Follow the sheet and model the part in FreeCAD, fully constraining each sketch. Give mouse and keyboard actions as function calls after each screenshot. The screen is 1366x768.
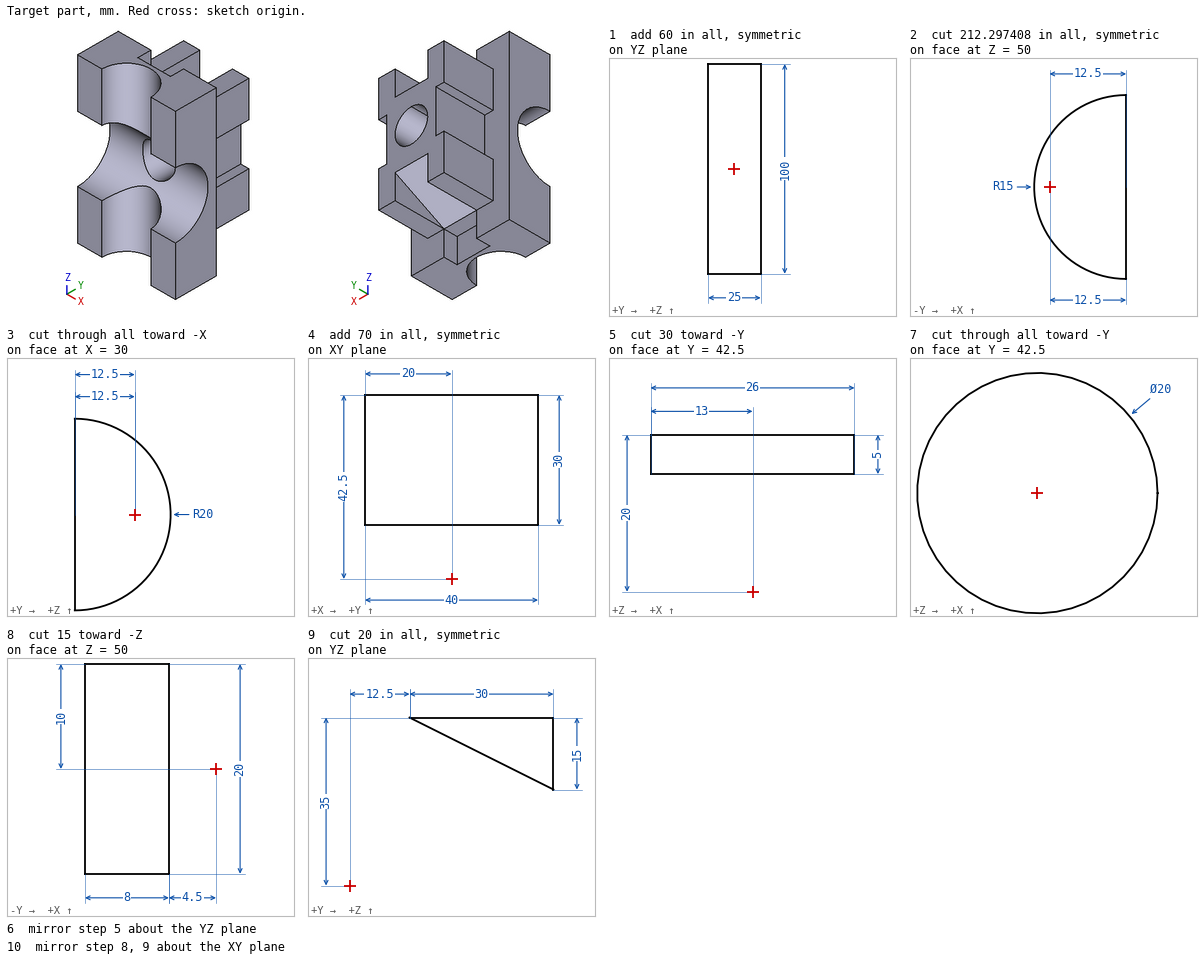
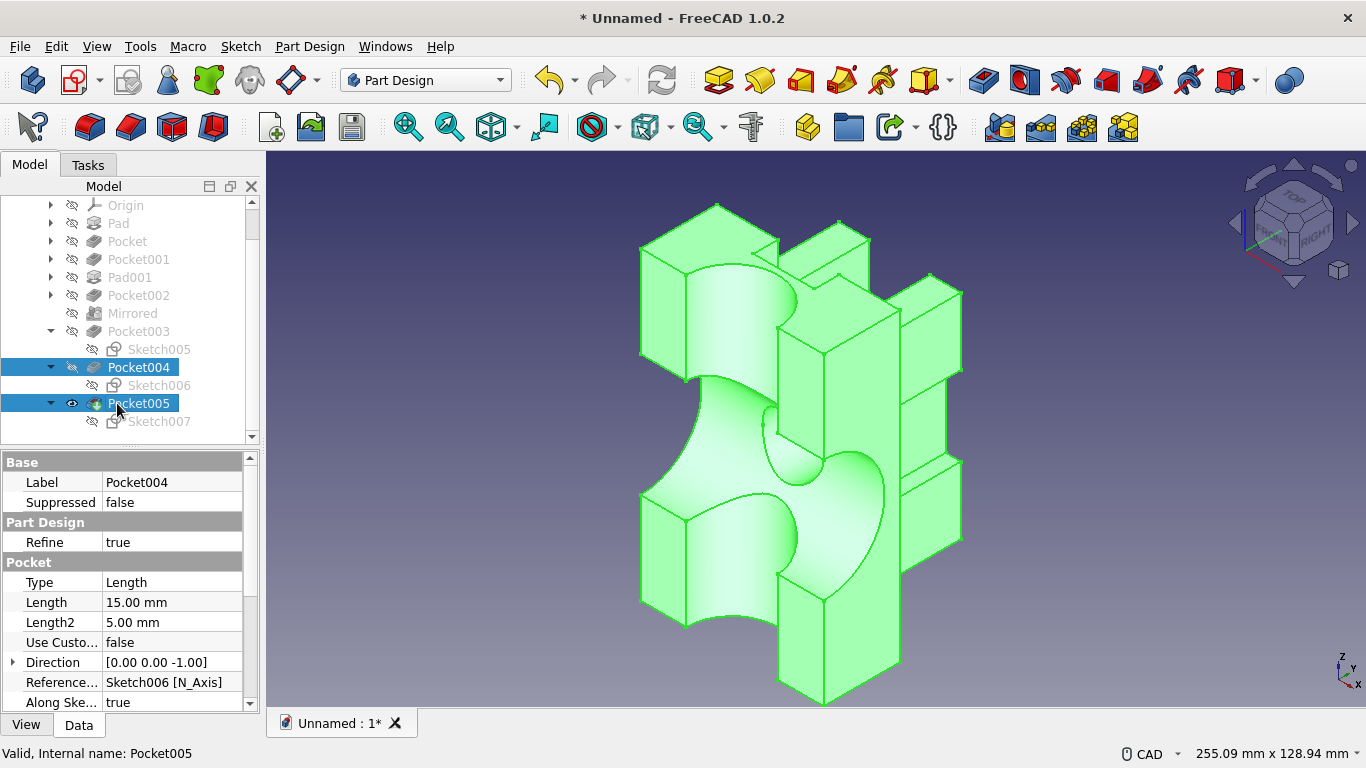
click(1000, 128)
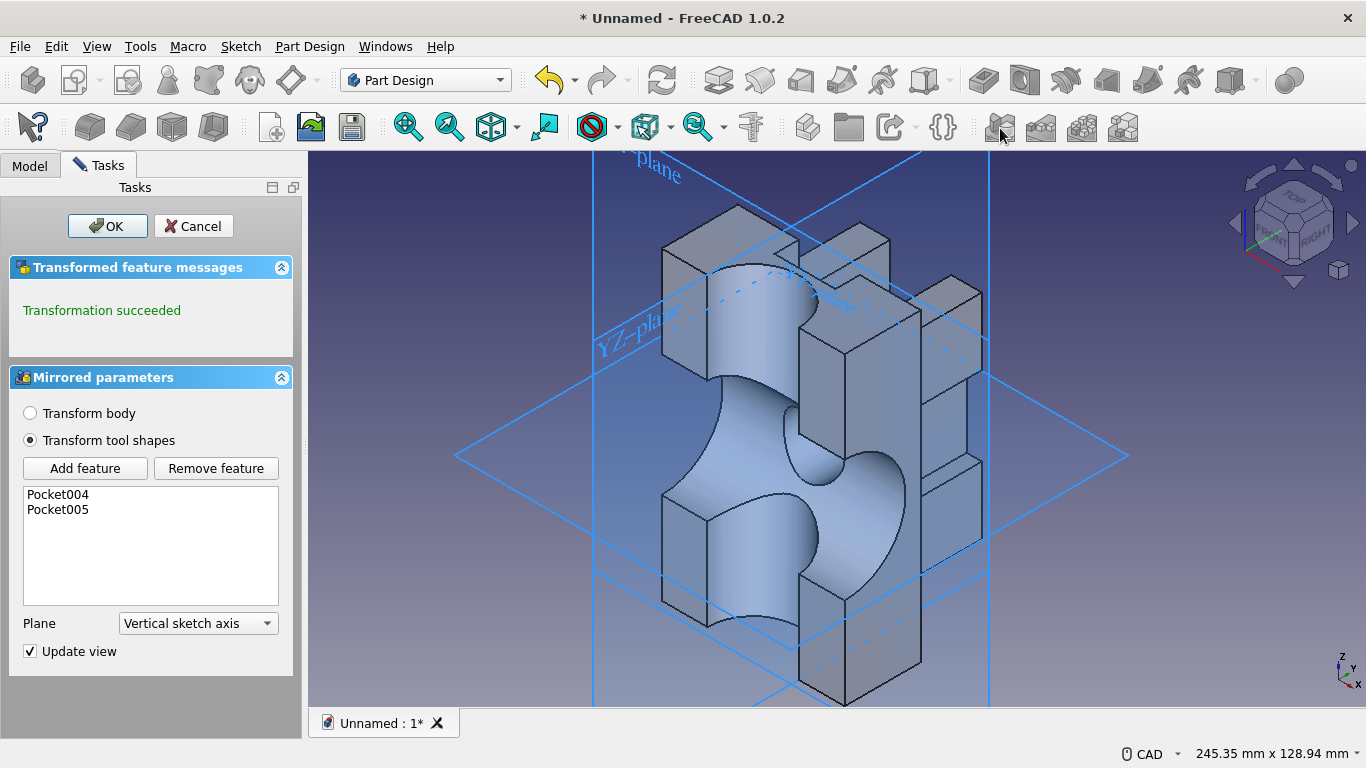
click(199, 624)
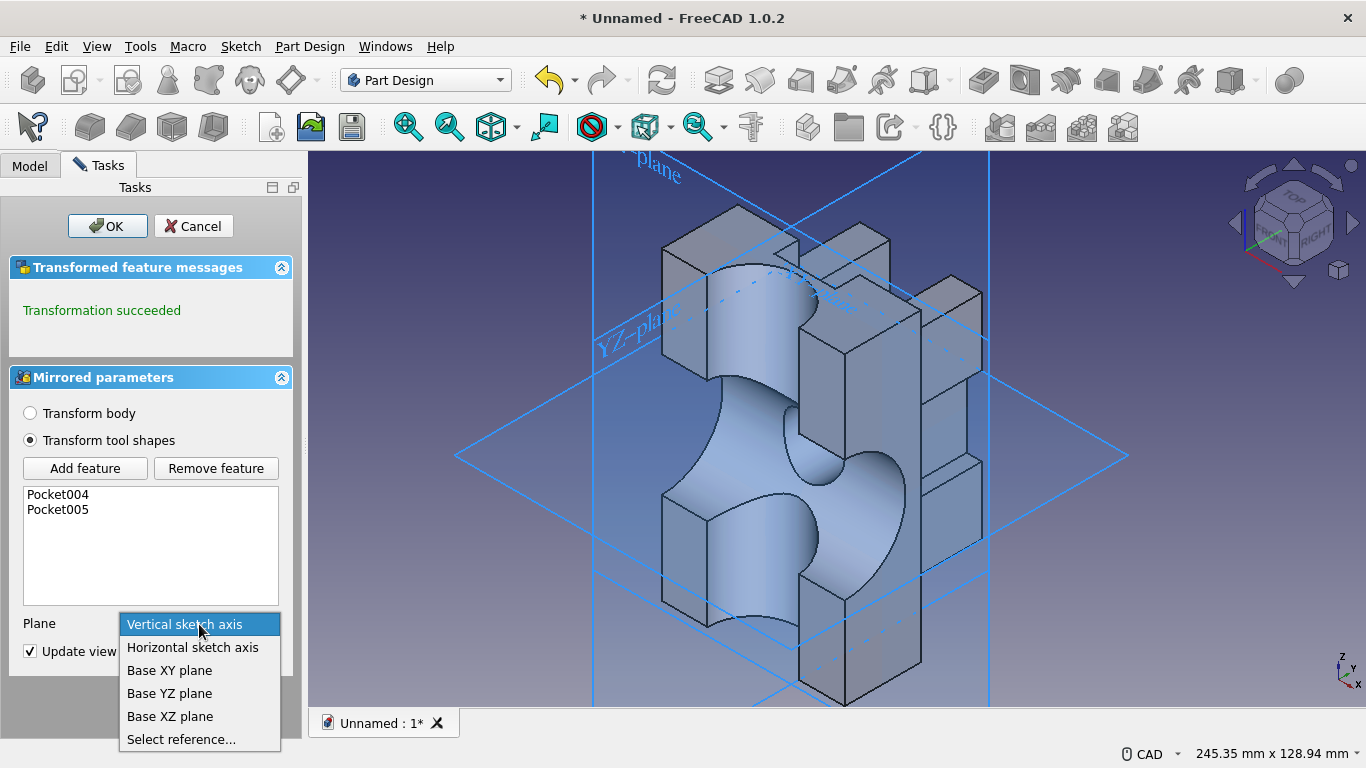
click(198, 670)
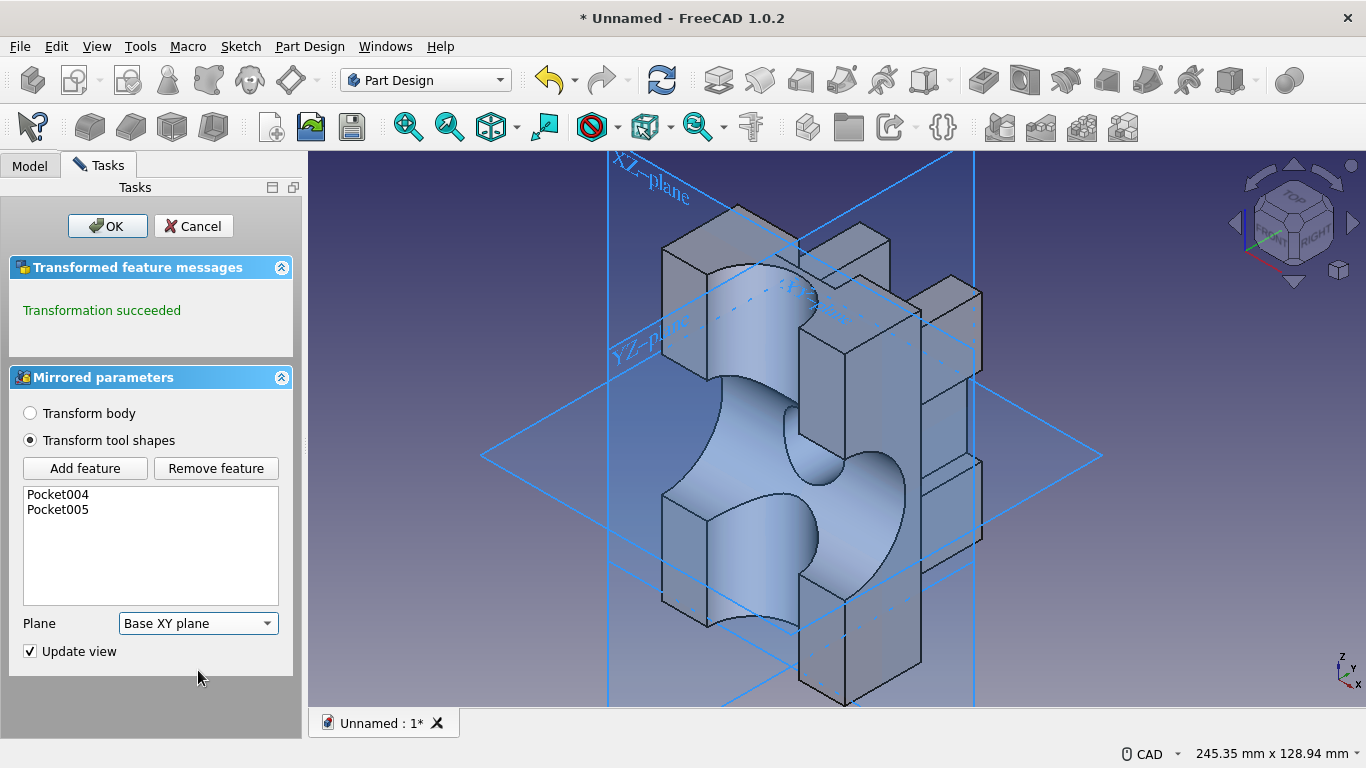
click(108, 226)